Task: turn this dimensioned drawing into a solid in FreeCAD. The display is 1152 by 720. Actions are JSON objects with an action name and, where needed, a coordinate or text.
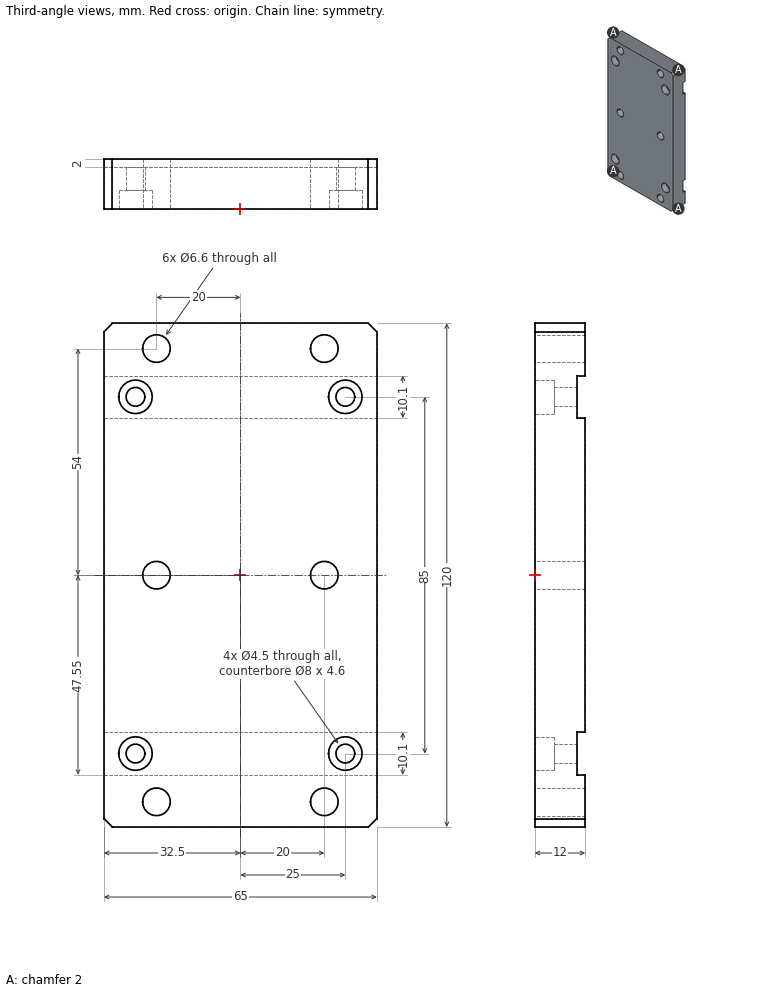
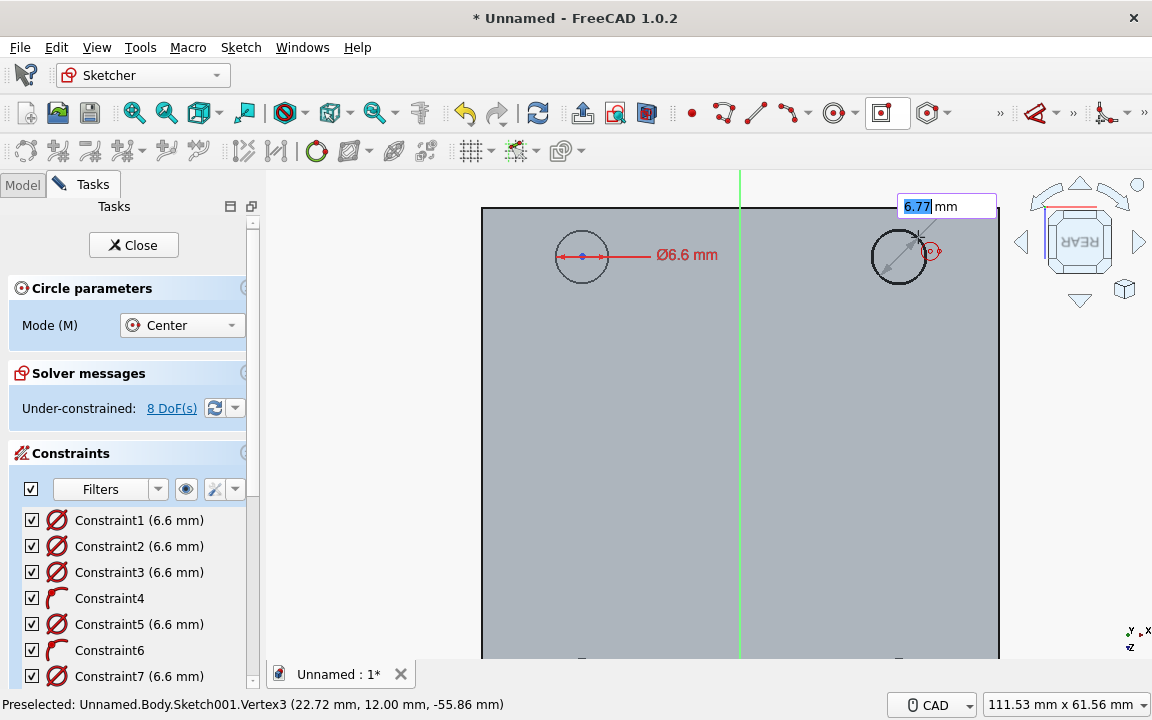
{"action": "type", "text": "6.6"}
{"action": "key", "text": "Return"}
{"action": "key", "text": "Escape"}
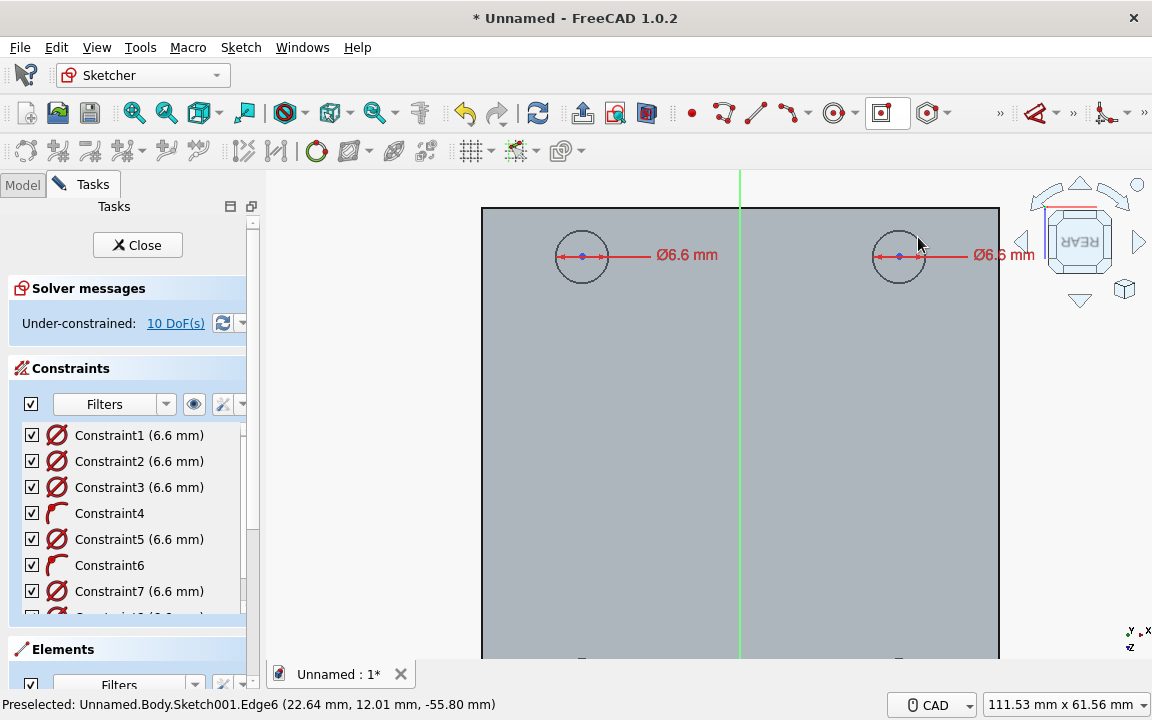
{"action": "scroll", "coordinate": [582, 257], "scroll_direction": "down", "scroll_amount": 5}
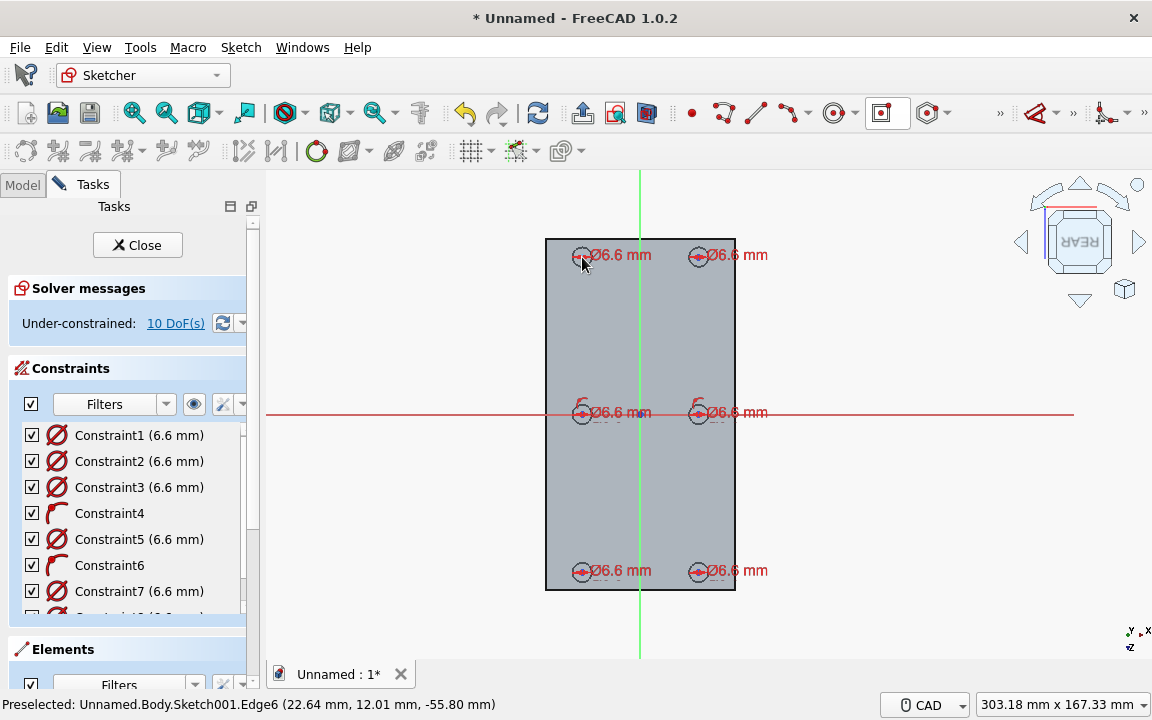
{"action": "left_click", "coordinate": [582, 573]}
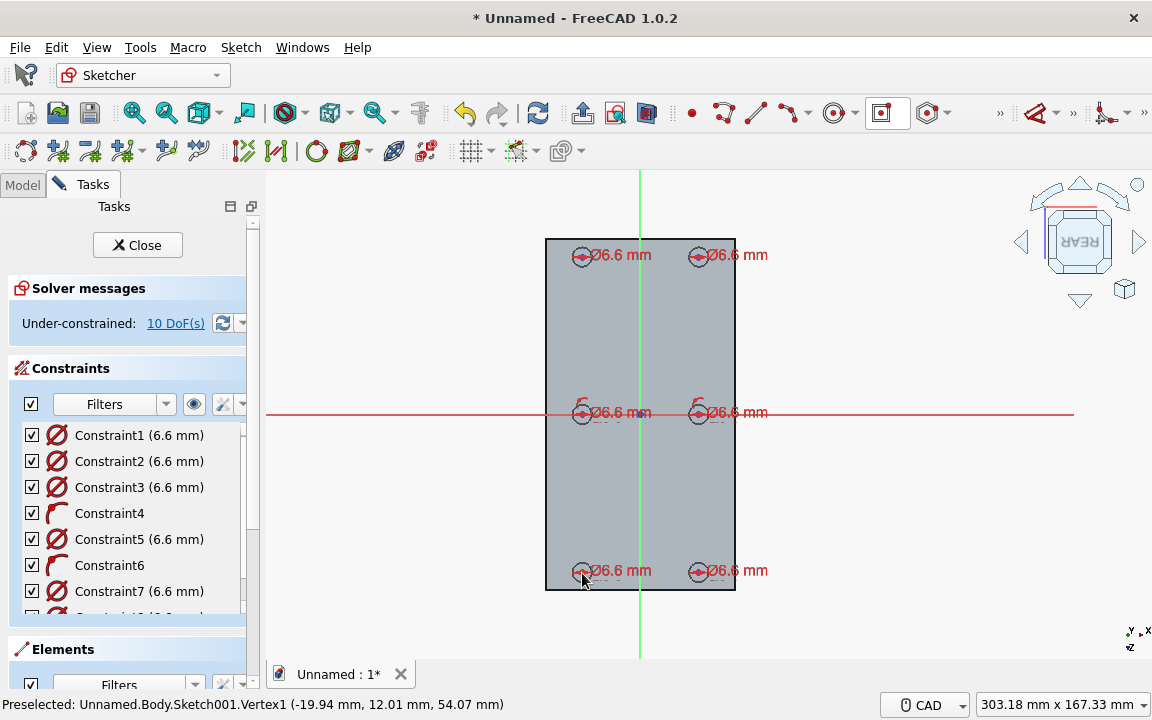
{"action": "left_click", "coordinate": [699, 573]}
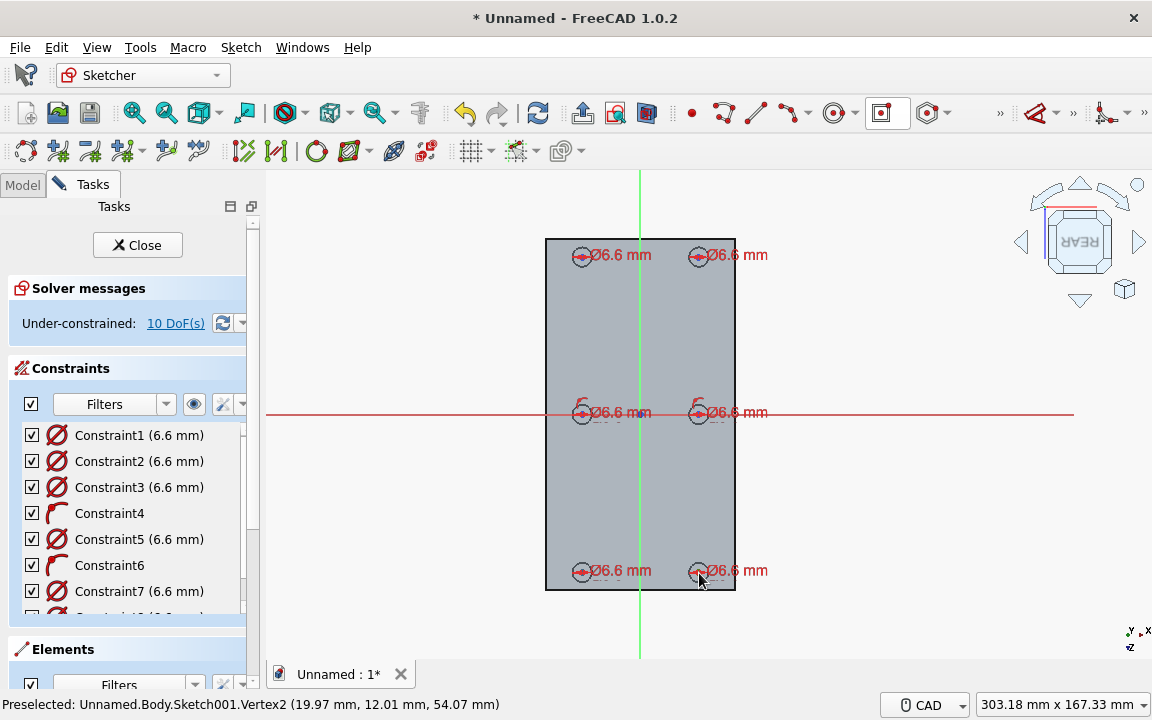
{"action": "left_click", "coordinate": [640, 600]}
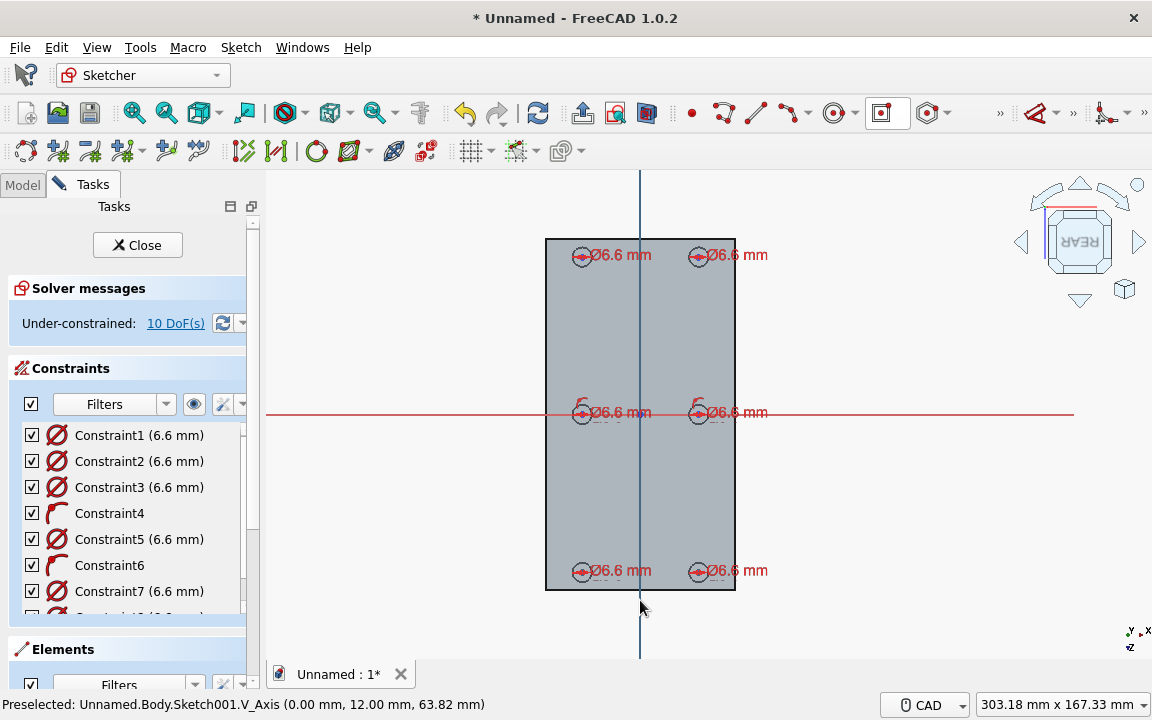
{"action": "key", "text": "s"}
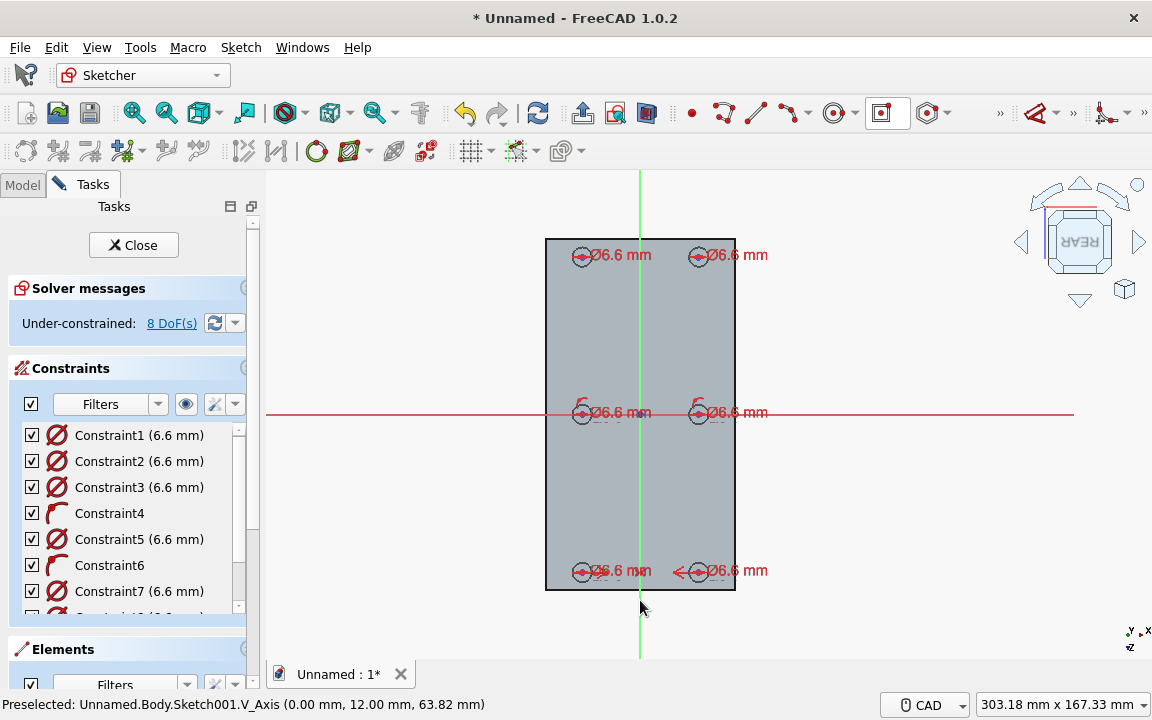
{"action": "left_click", "coordinate": [582, 573]}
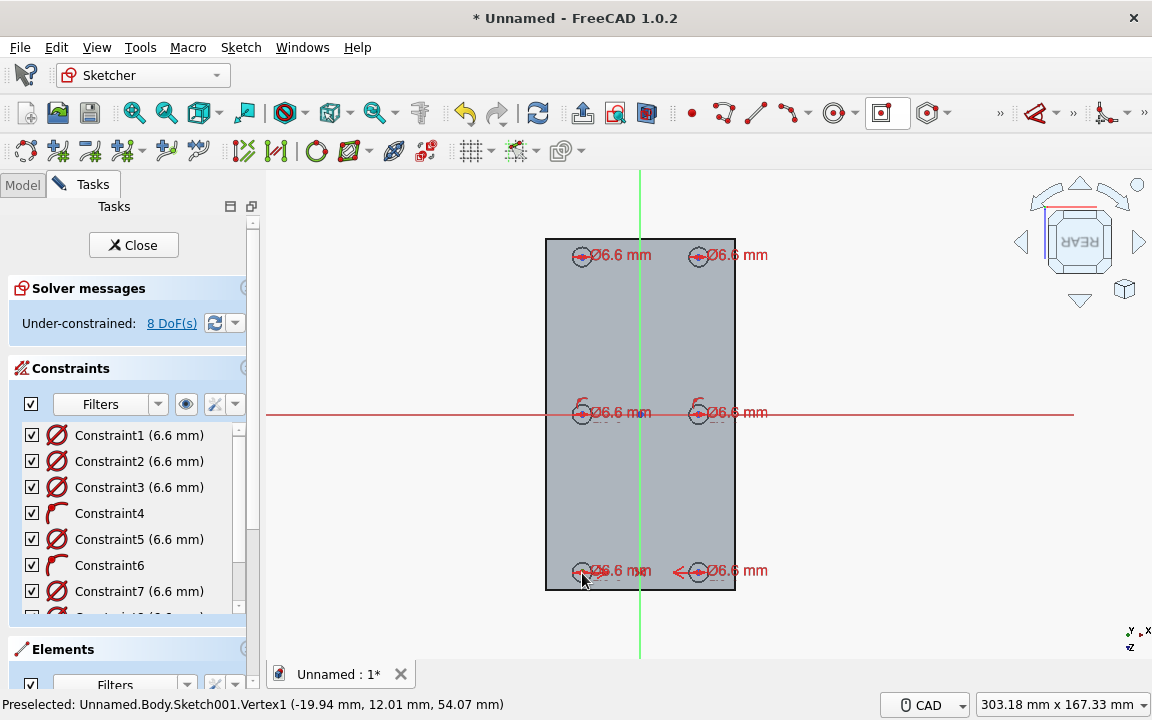
{"action": "left_click", "coordinate": [582, 257]}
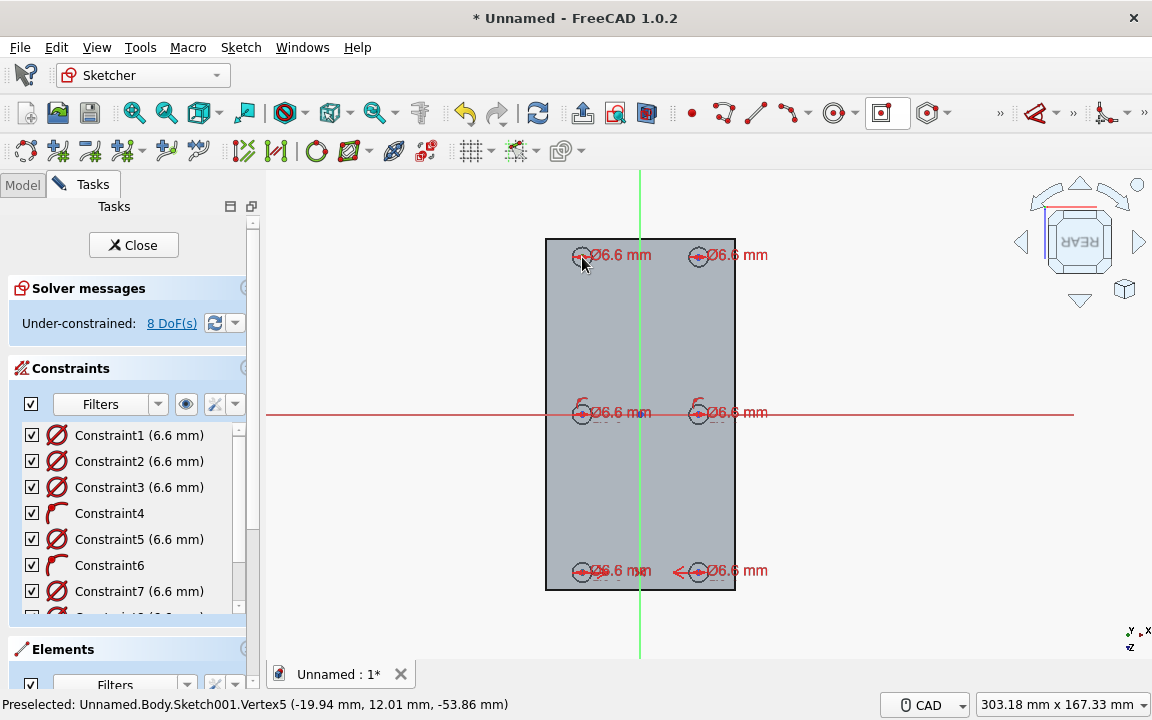
{"action": "left_click", "coordinate": [344, 414]}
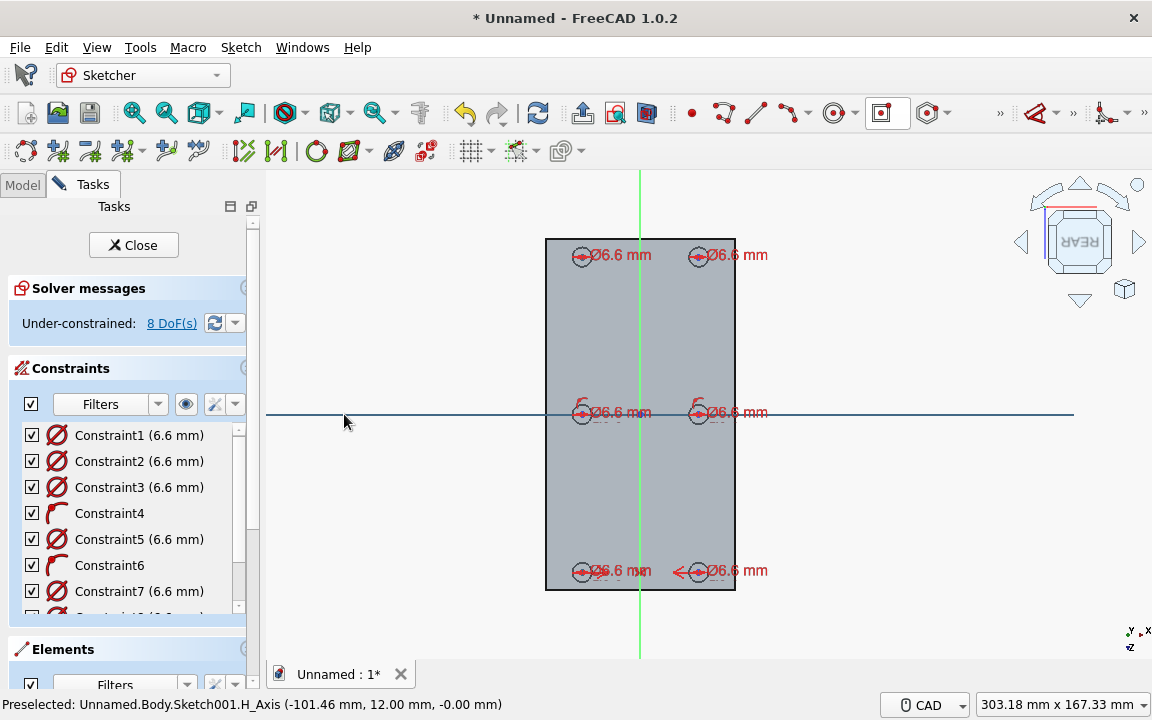
{"action": "key", "text": "s"}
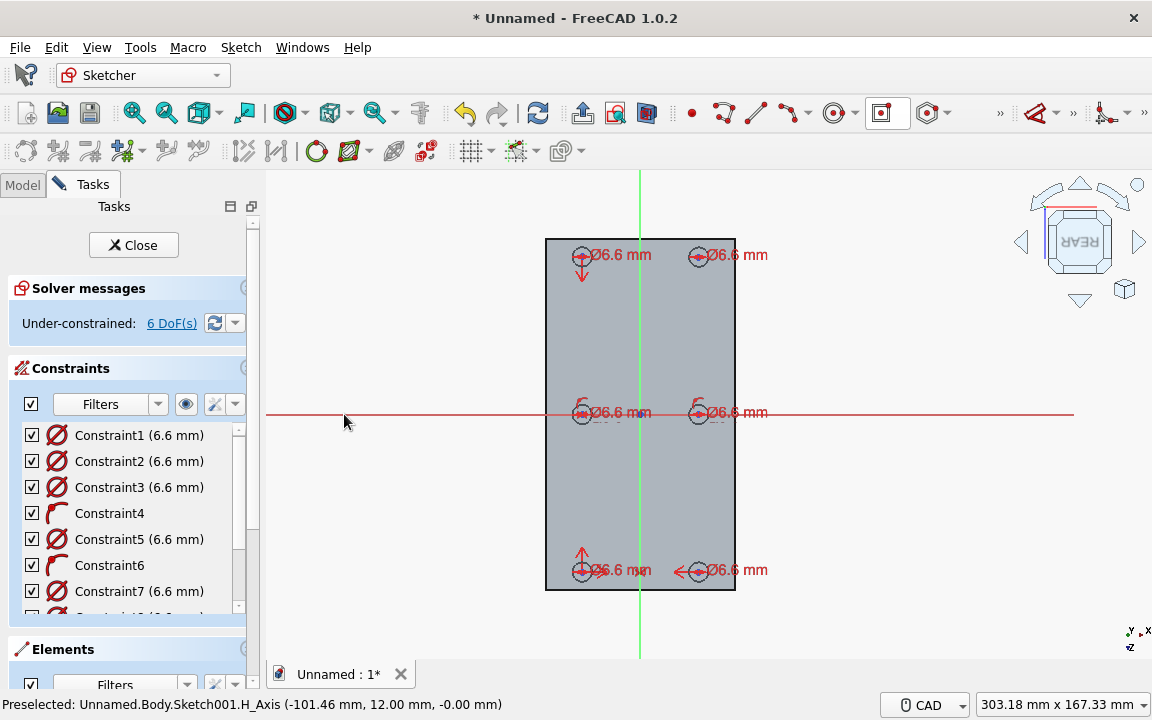
{"action": "left_click", "coordinate": [699, 572]}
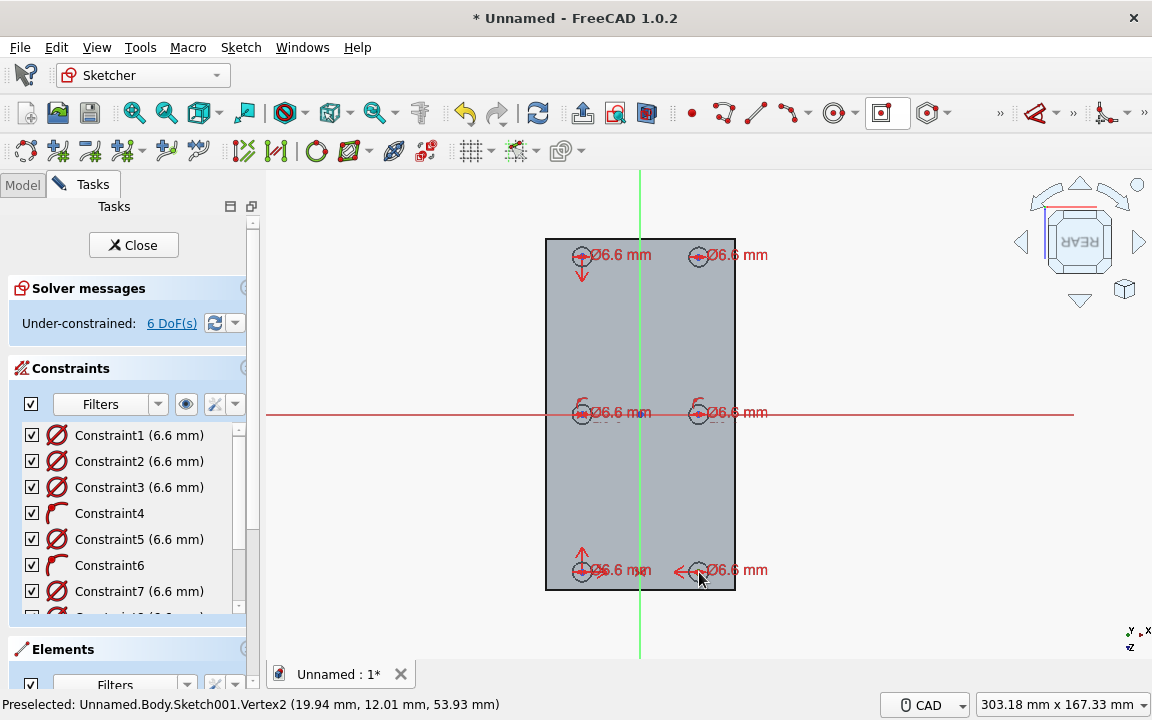
{"action": "left_click", "coordinate": [699, 257]}